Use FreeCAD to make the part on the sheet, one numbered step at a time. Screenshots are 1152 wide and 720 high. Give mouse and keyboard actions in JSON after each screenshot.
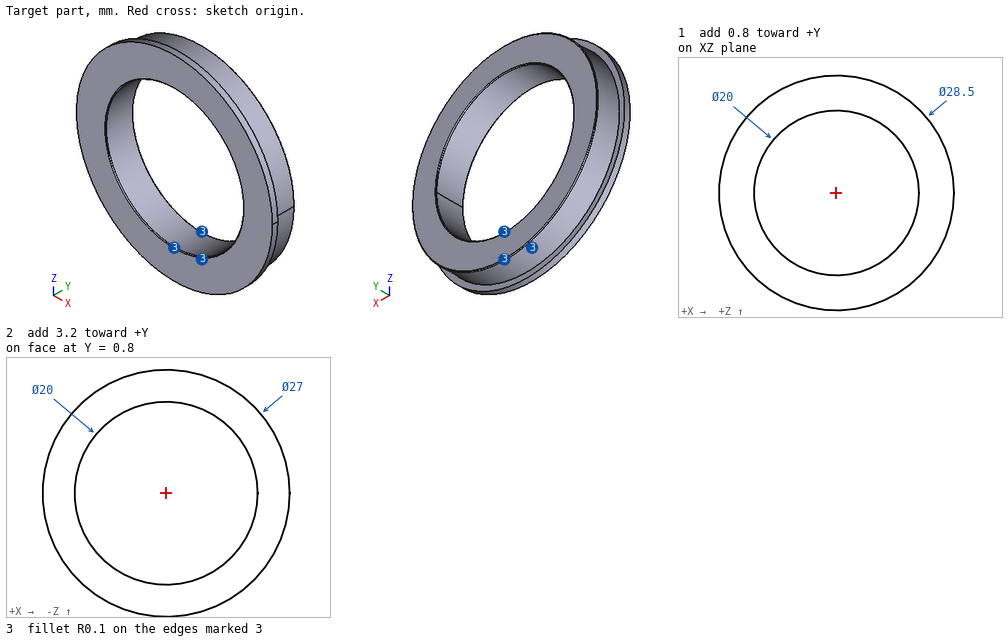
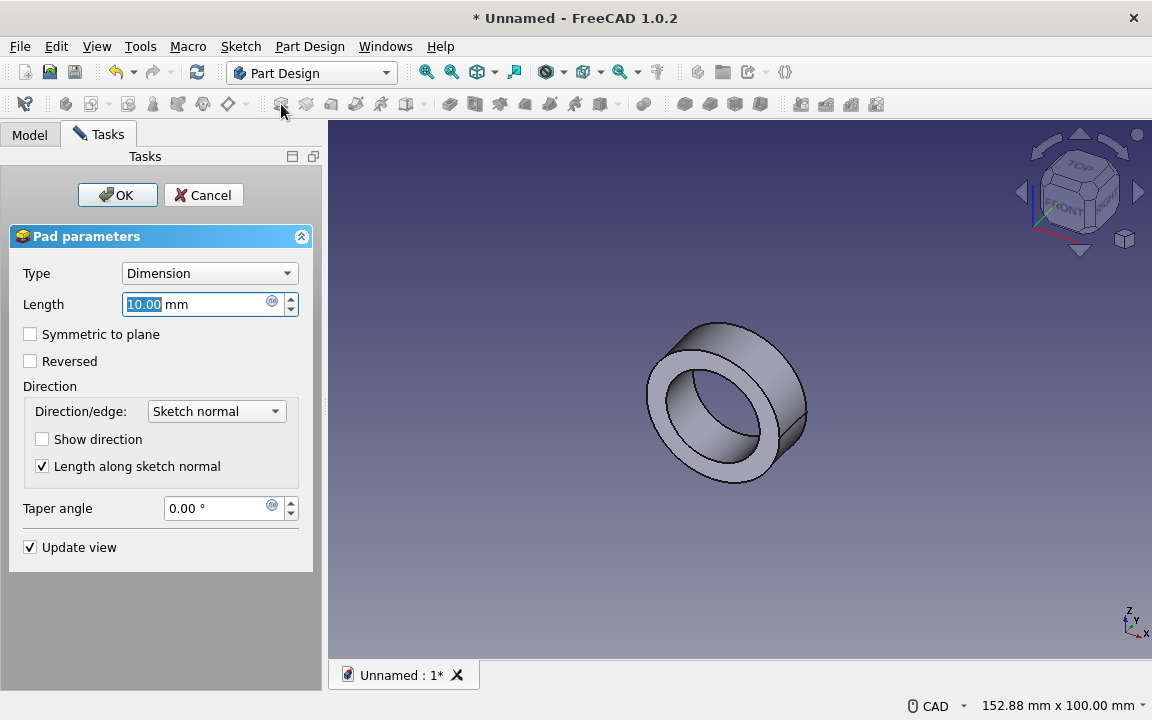
{"action": "type", "text": "0.8"}
{"action": "key", "text": "Tab"}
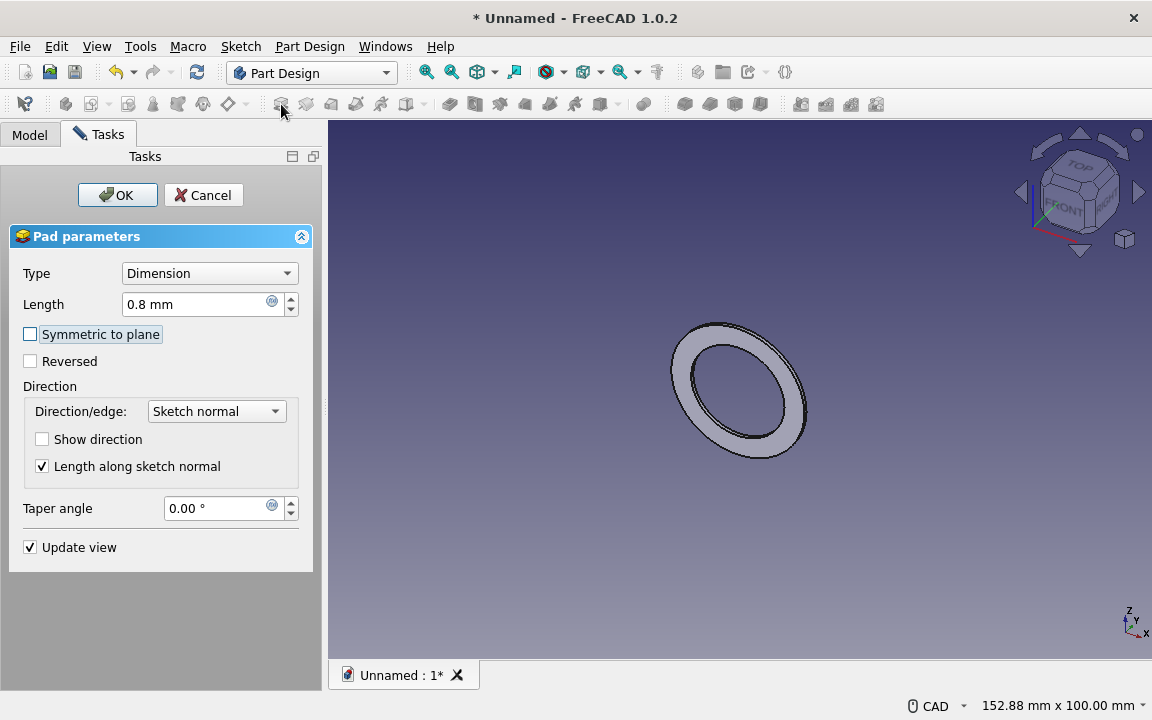
{"action": "left_click", "coordinate": [31, 361]}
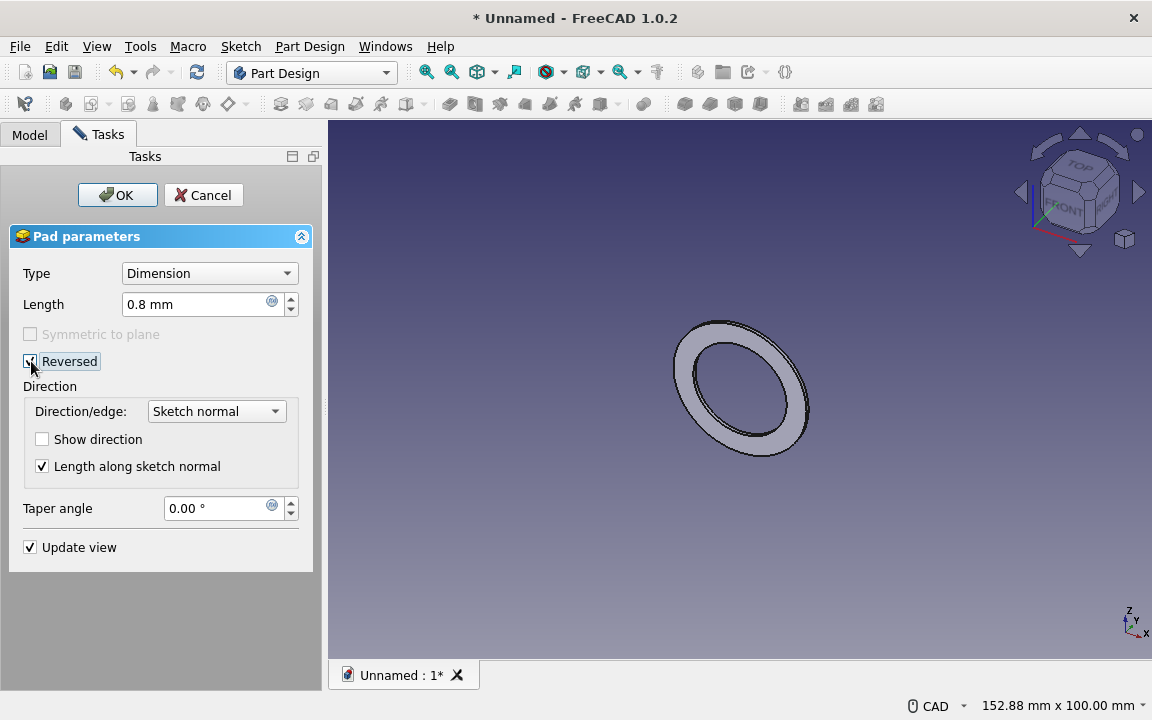
{"action": "left_click", "coordinate": [118, 195]}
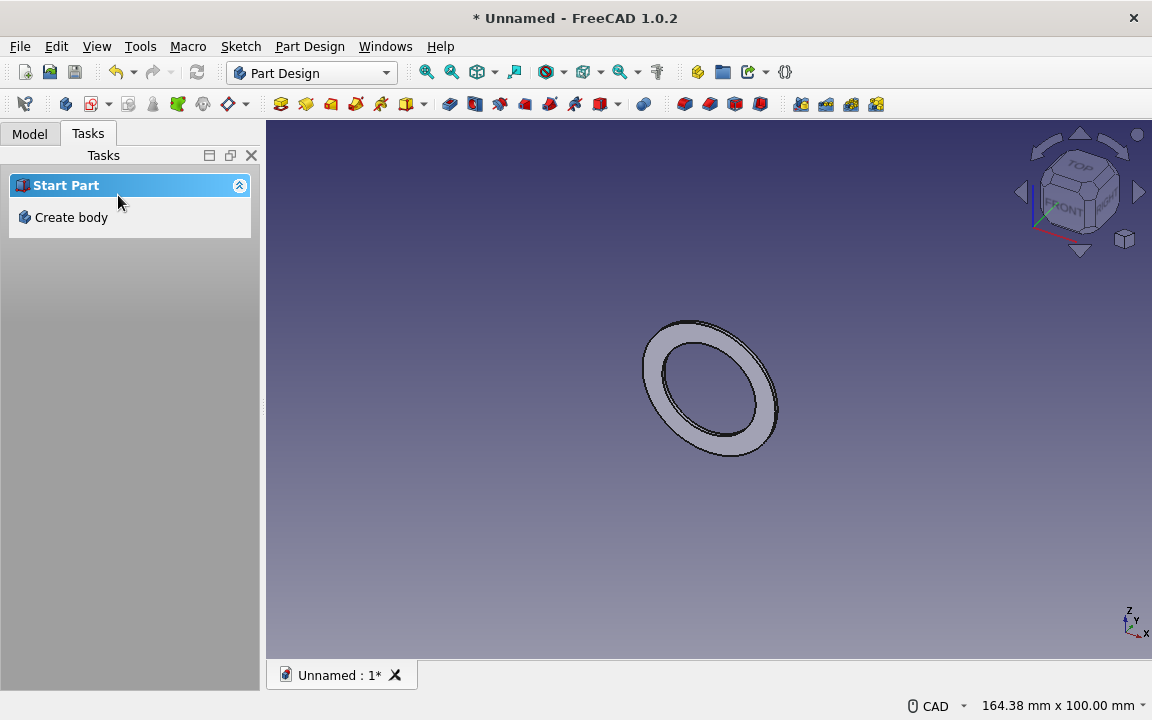
{"action": "key", "text": "v f"}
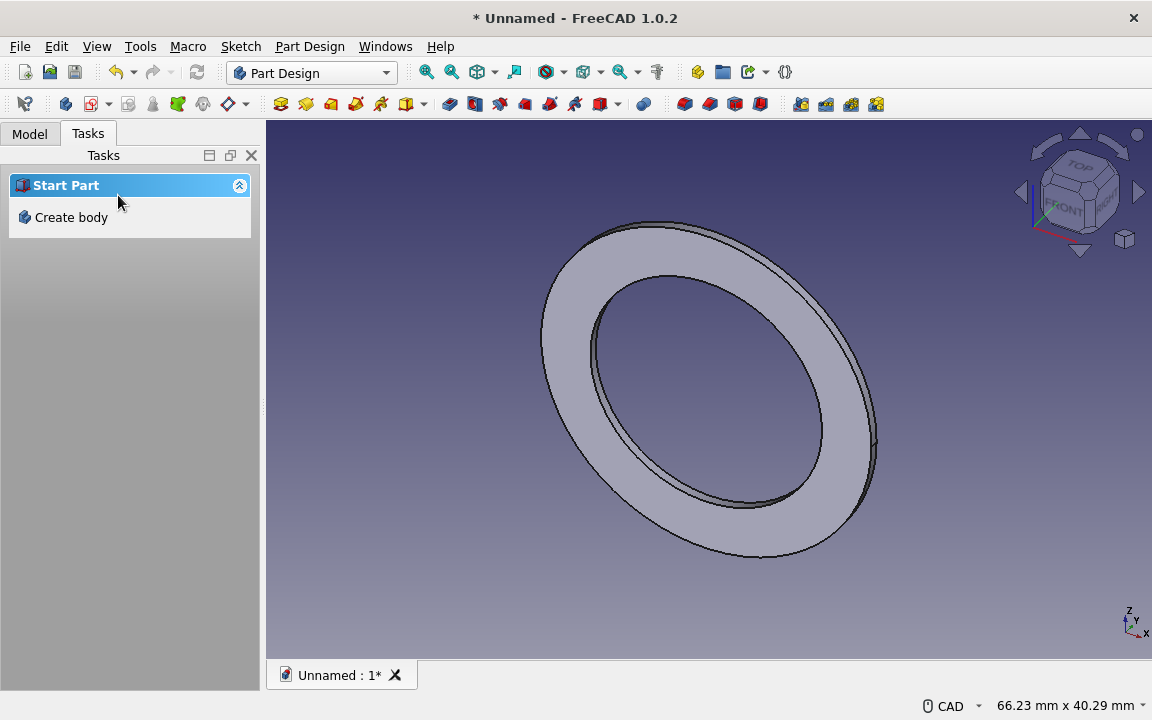
{"action": "key", "text": "4"}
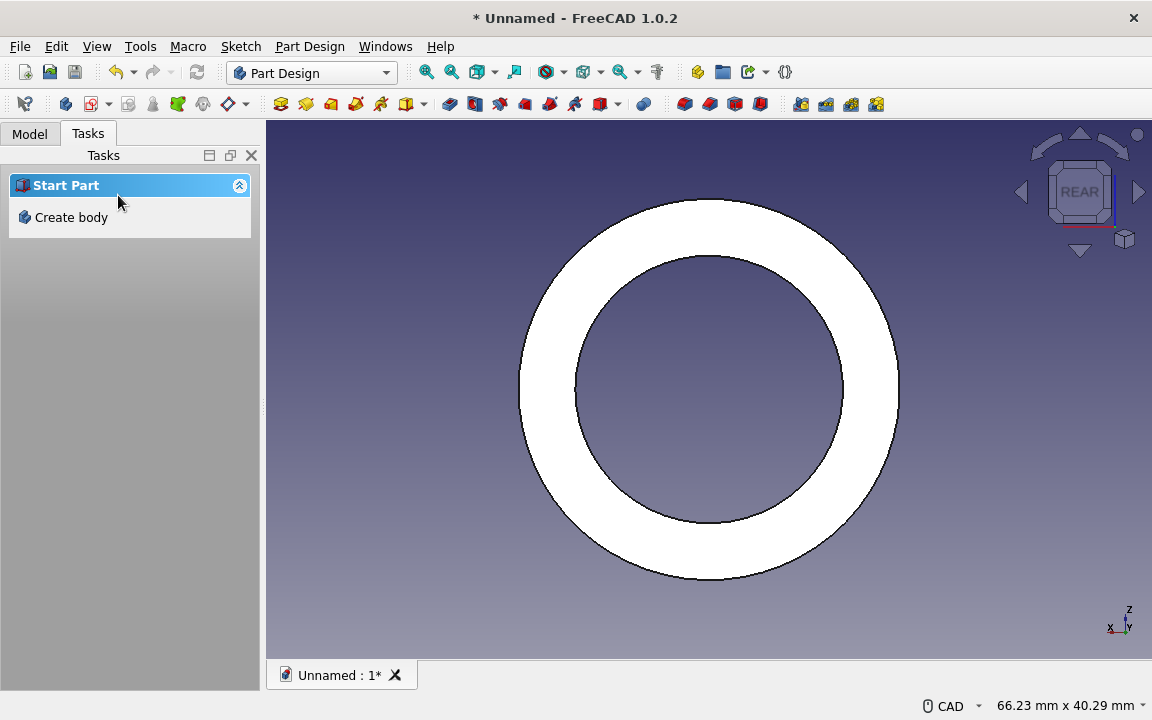
{"action": "left_click", "coordinate": [873, 388]}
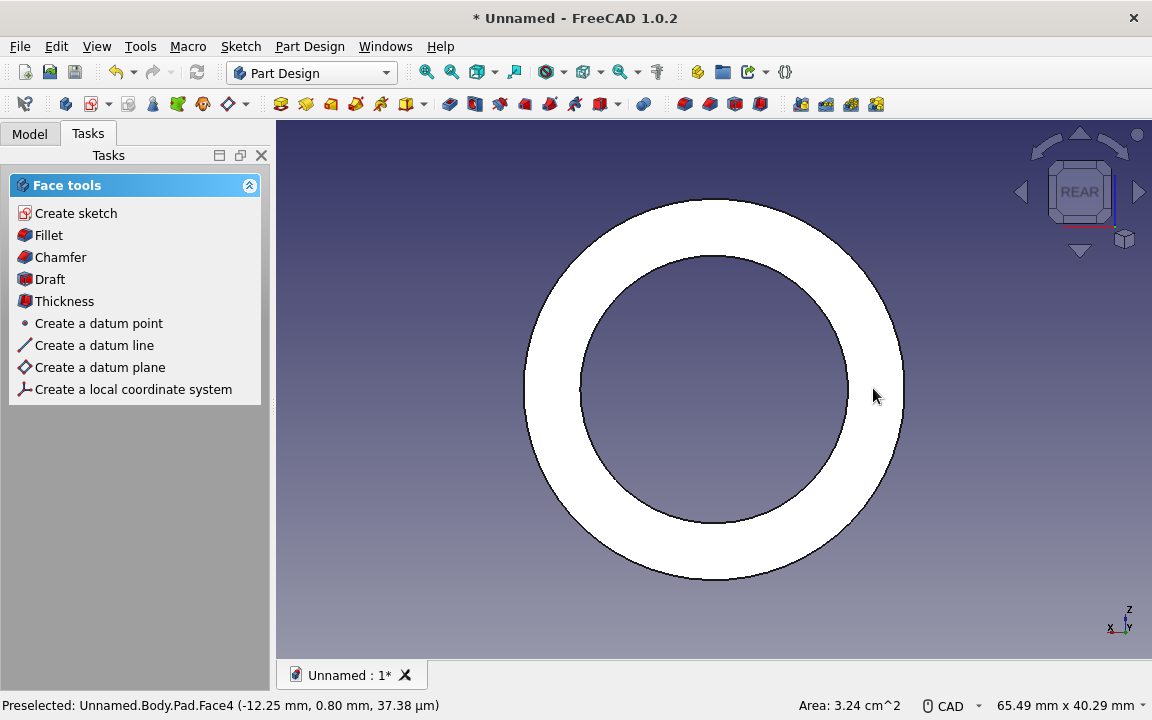
{"action": "left_click", "coordinate": [90, 104]}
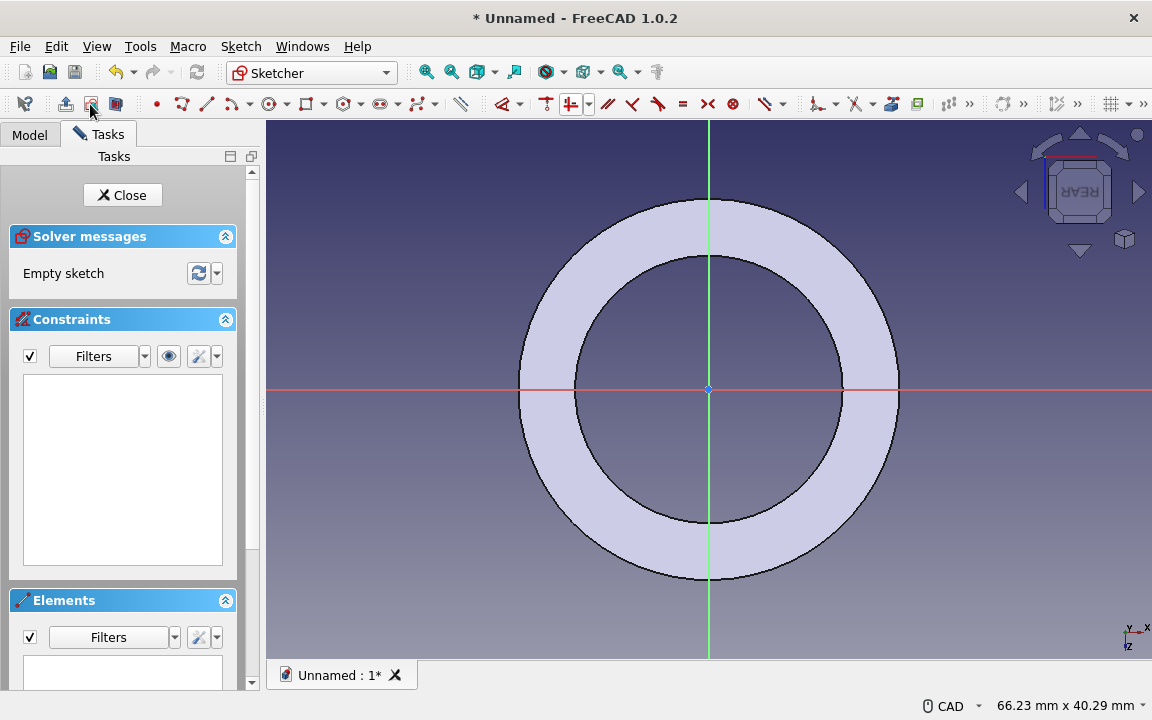
{"action": "key", "text": "g c"}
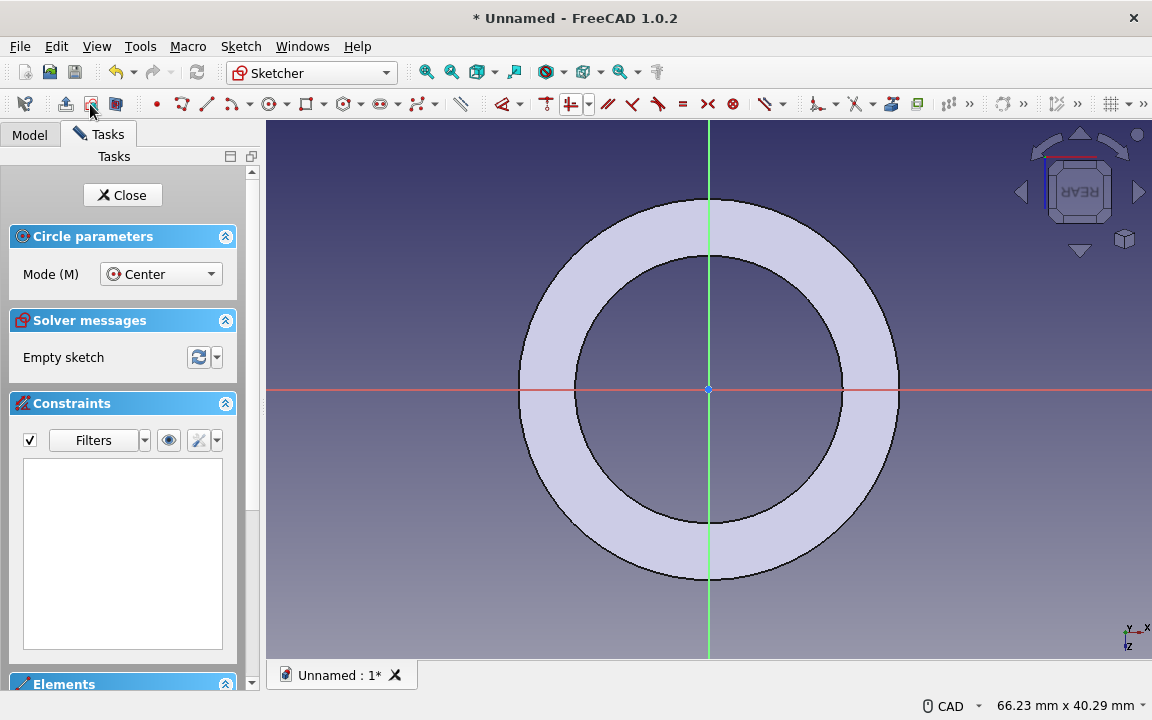
{"action": "left_click", "coordinate": [709, 390]}
{"action": "mouse_move", "coordinate": [837, 262]}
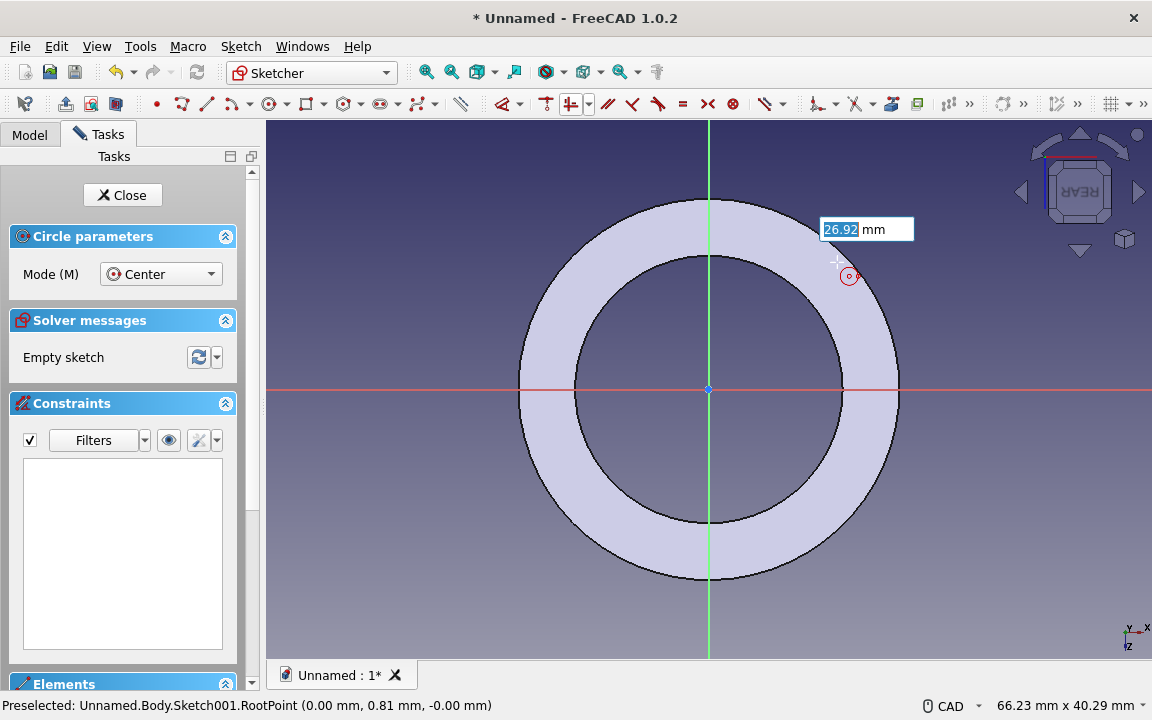
{"action": "type", "text": "27"}
{"action": "key", "text": "Return"}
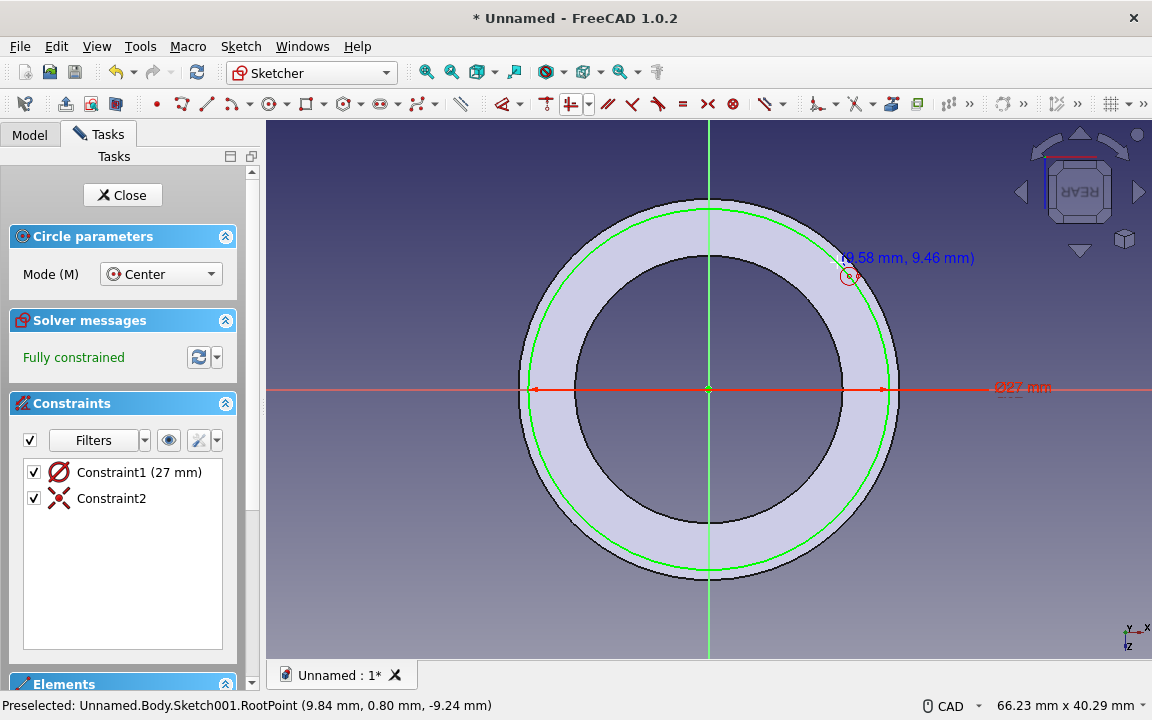
{"action": "left_click", "coordinate": [709, 390]}
{"action": "mouse_move", "coordinate": [803, 295]}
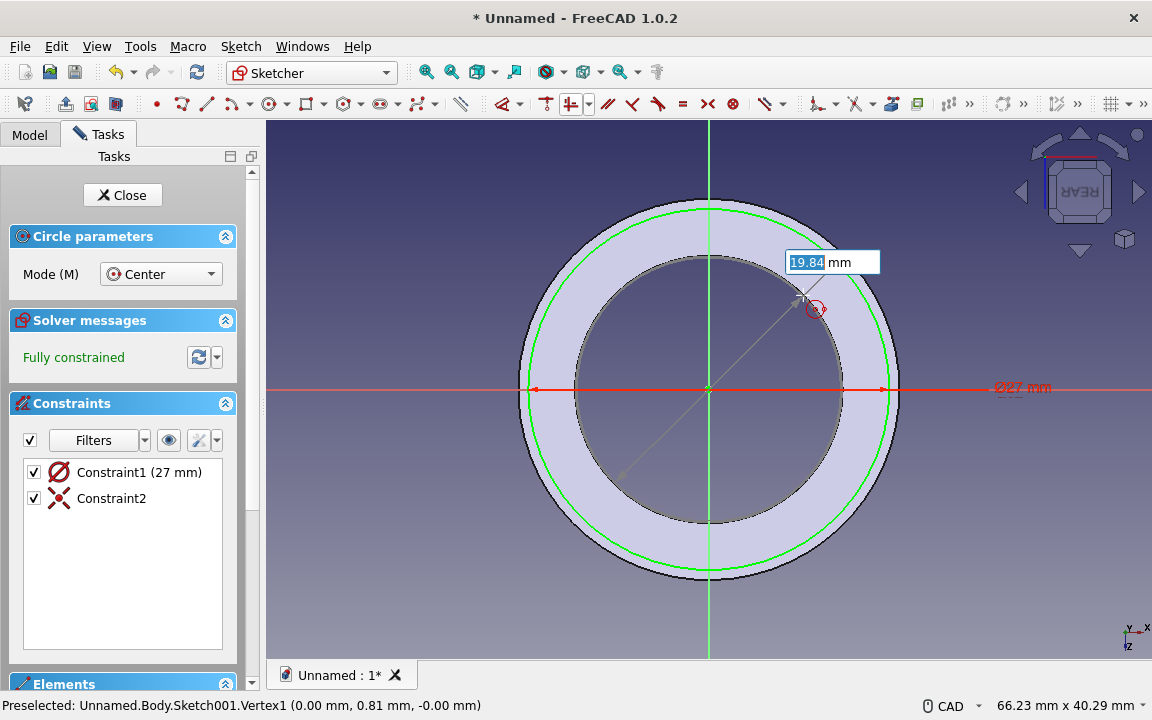
{"action": "type", "text": "20"}
{"action": "key", "text": "Return"}
{"action": "key", "text": "Escape"}